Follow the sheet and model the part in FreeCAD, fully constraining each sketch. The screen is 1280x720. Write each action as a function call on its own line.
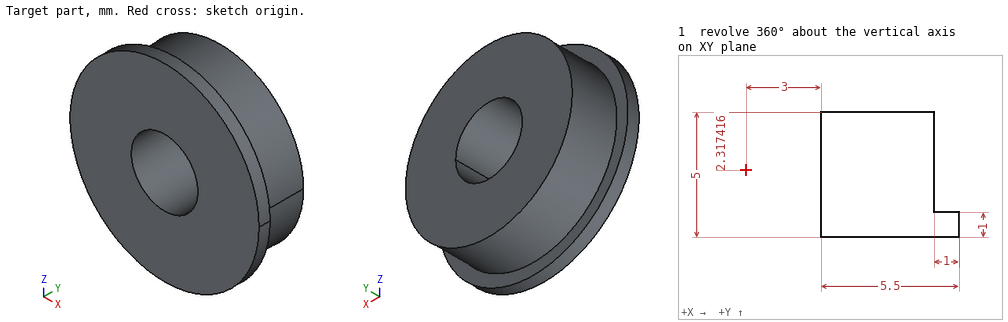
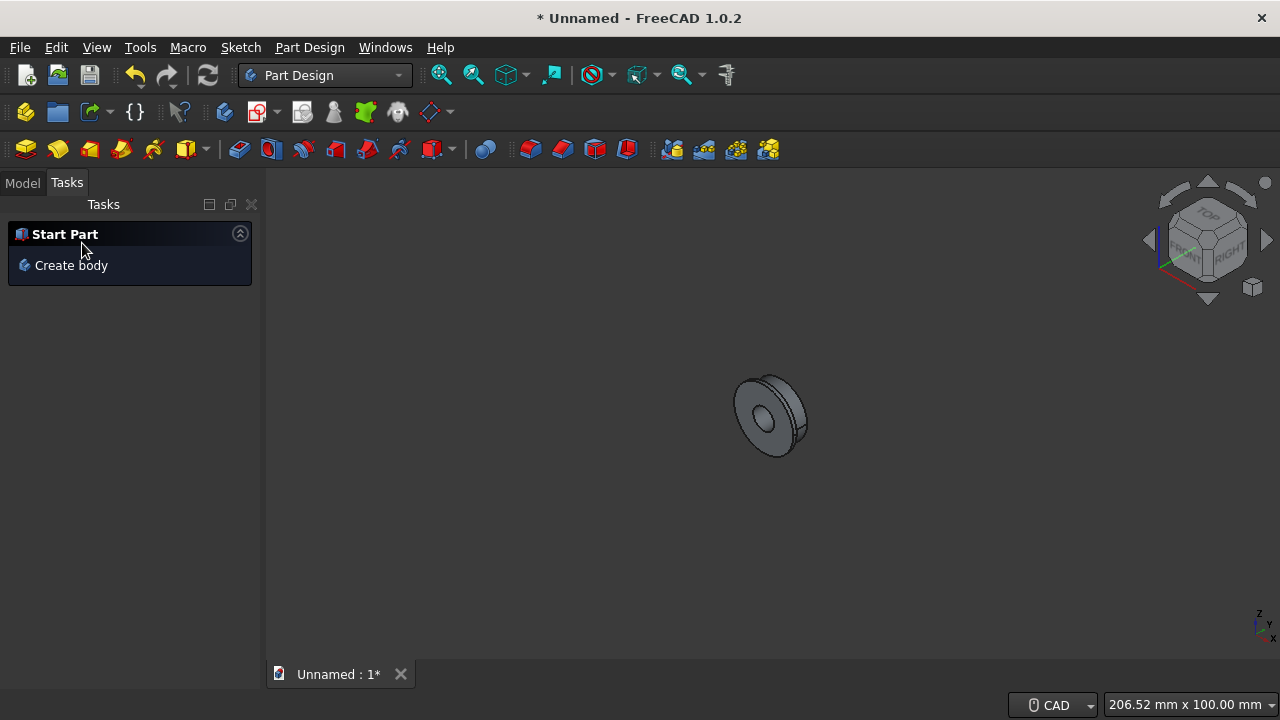
click(442, 76)